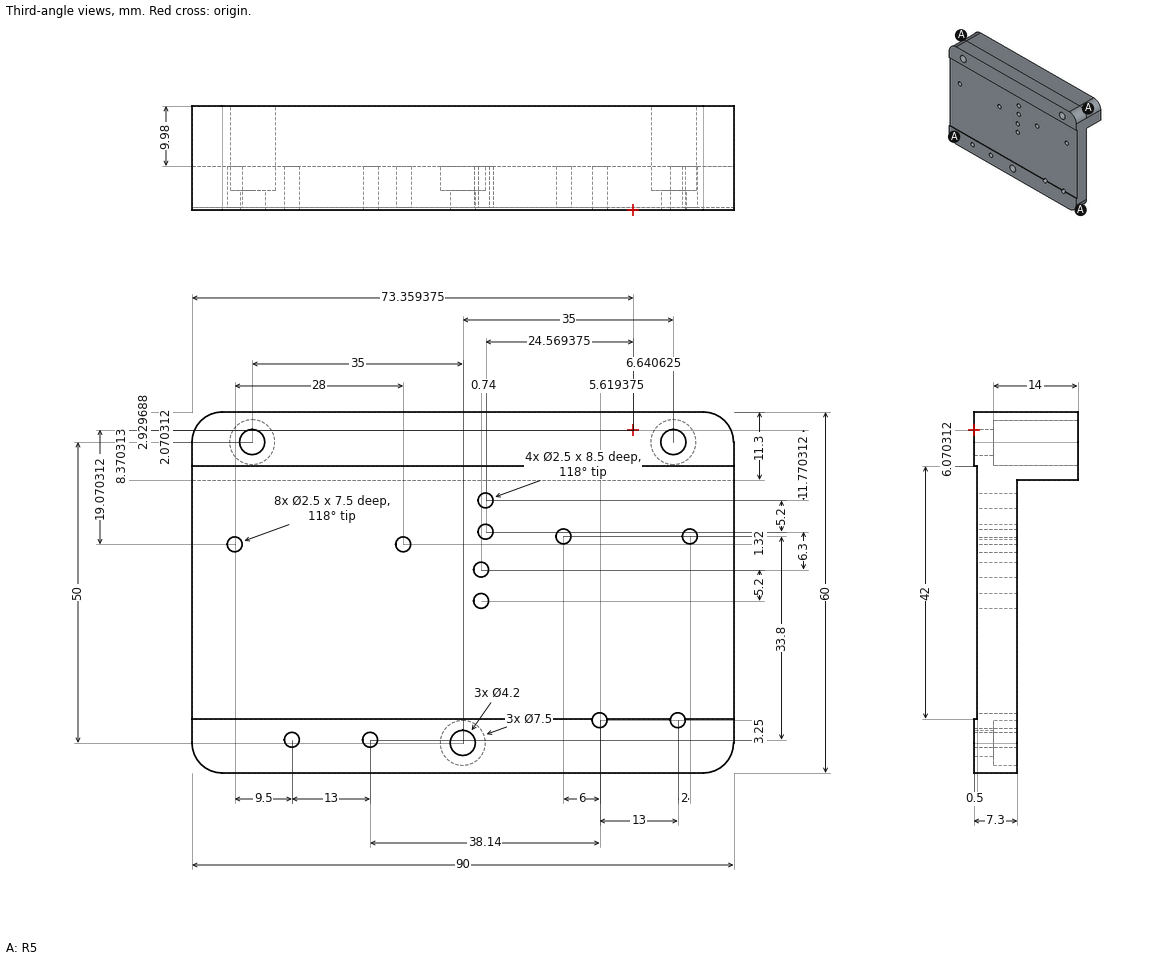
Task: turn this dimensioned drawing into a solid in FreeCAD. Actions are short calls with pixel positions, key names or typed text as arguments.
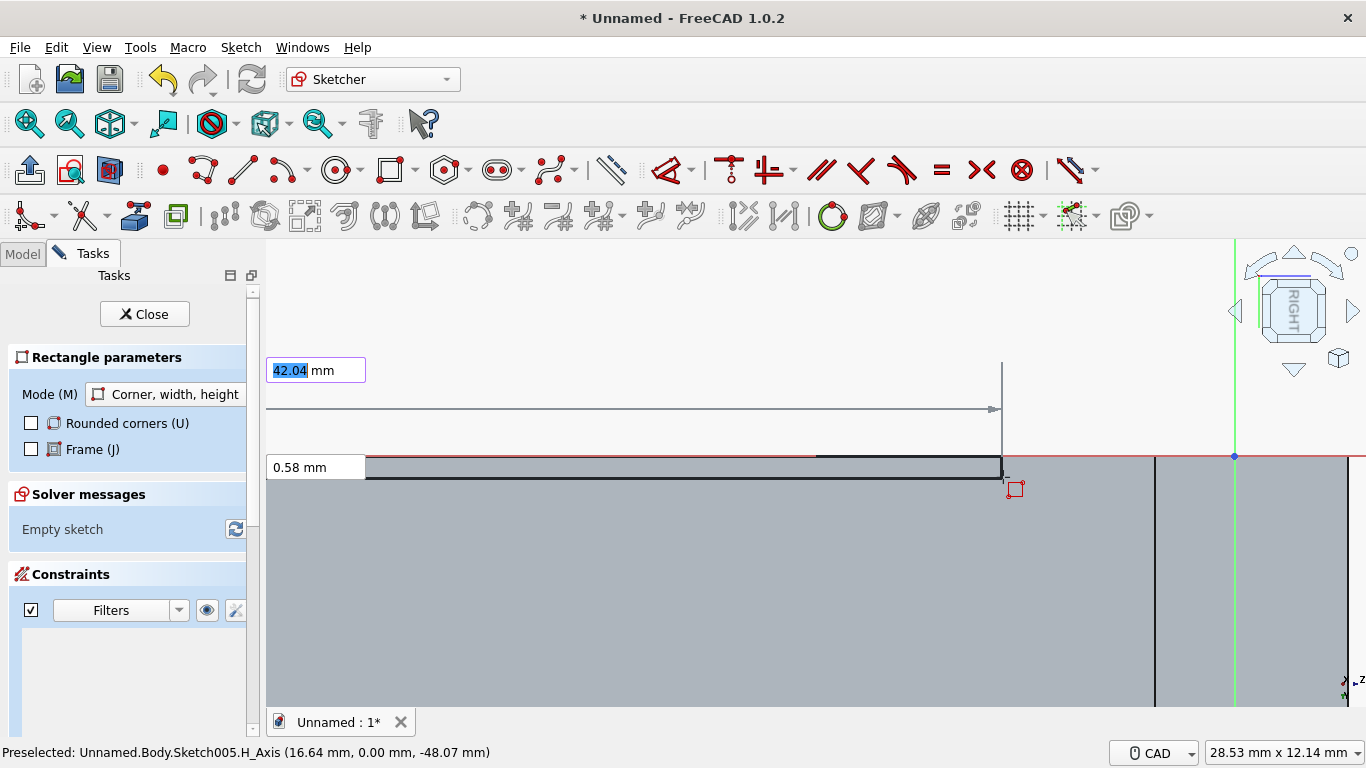
click(1001, 476)
key(Escape)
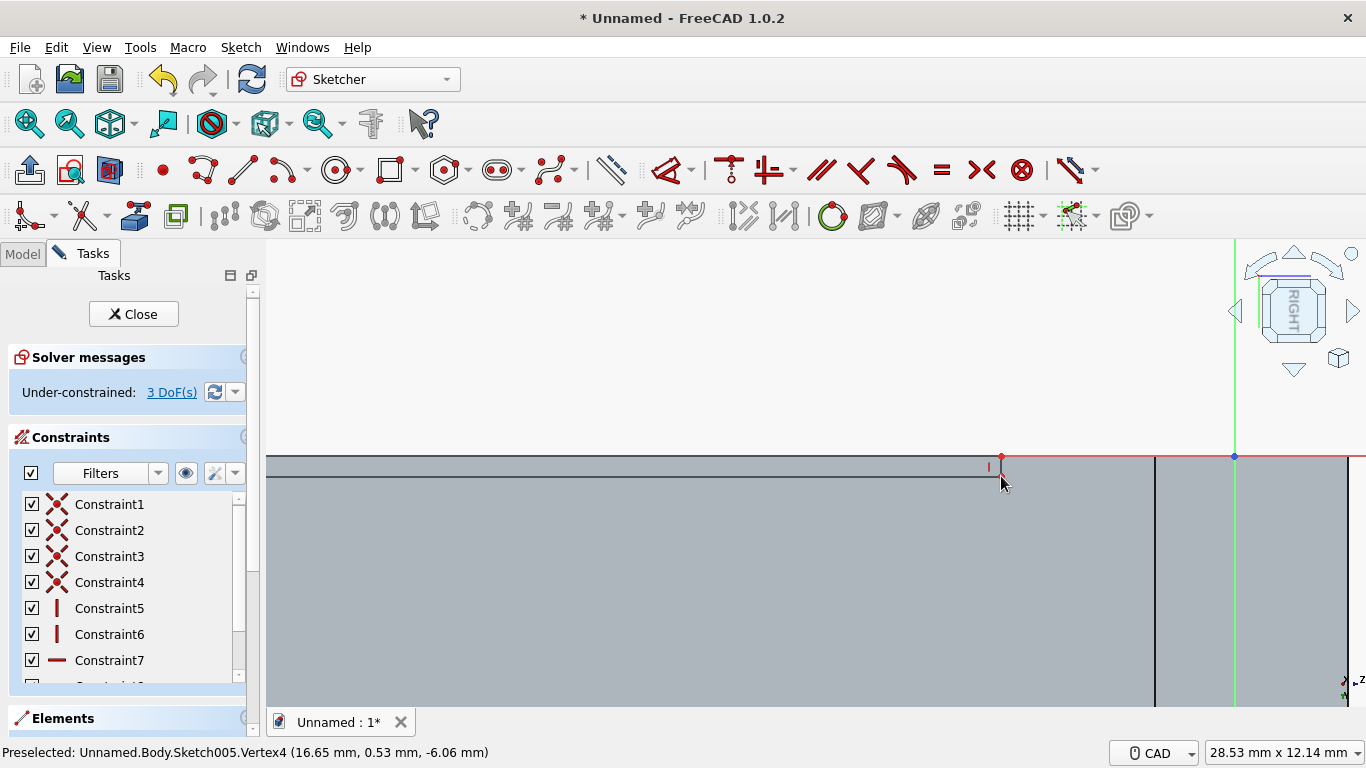
click(666, 170)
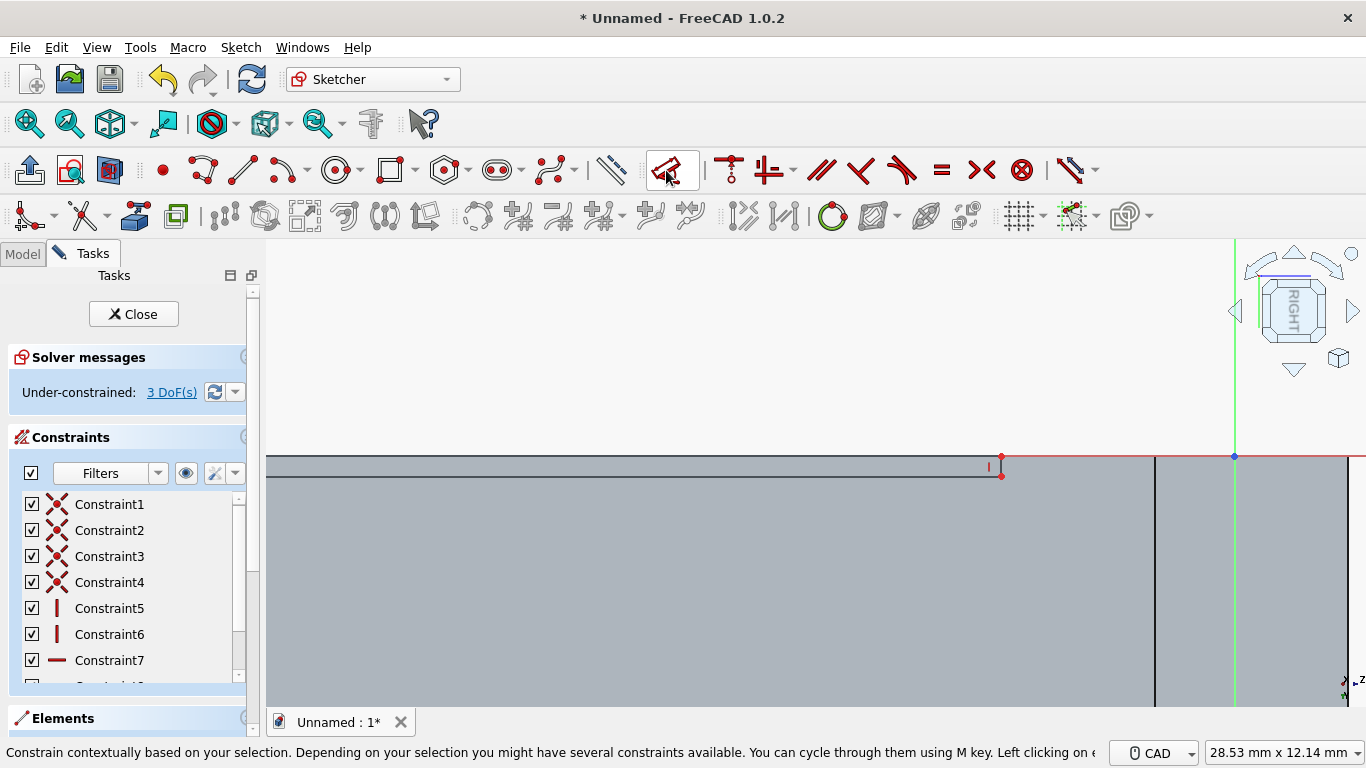
click(515, 477)
click(648, 511)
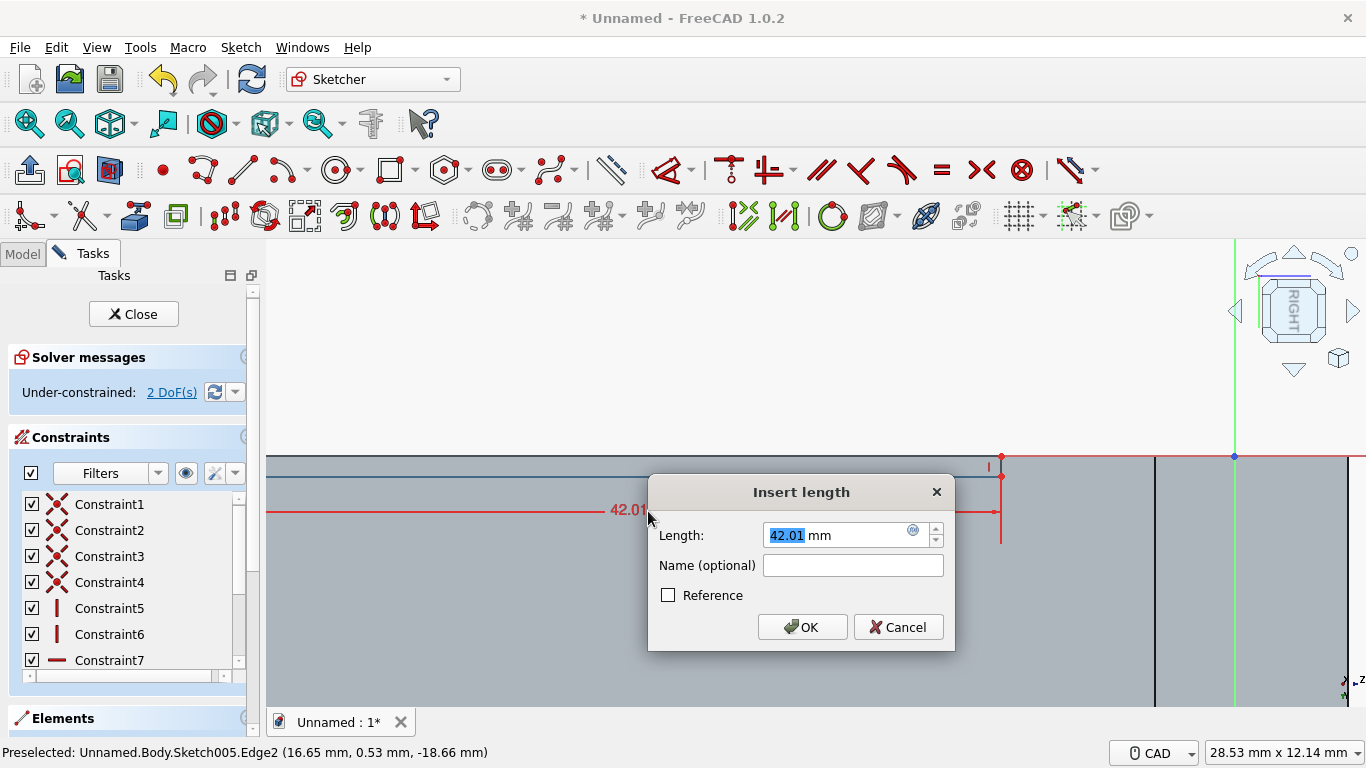
text(42)
key(Return)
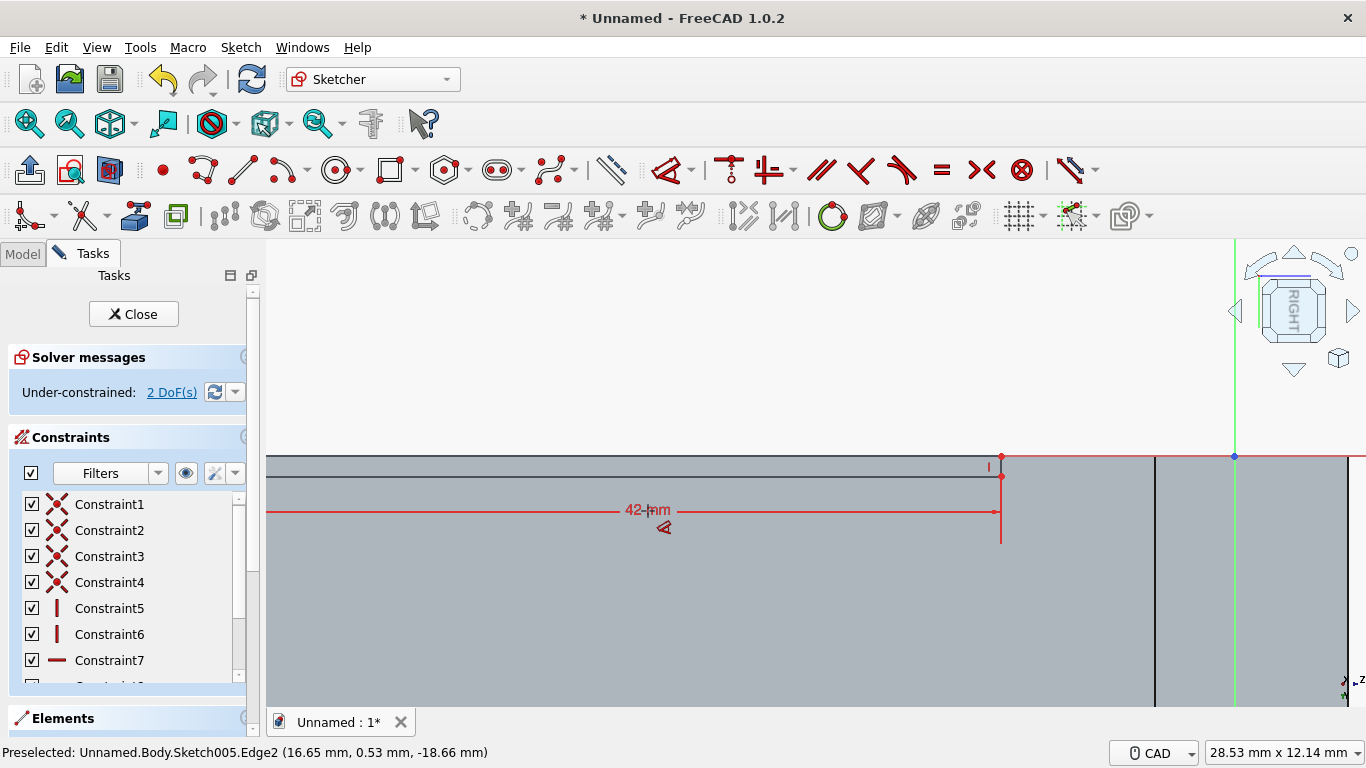
scroll(1003, 477, down, 5)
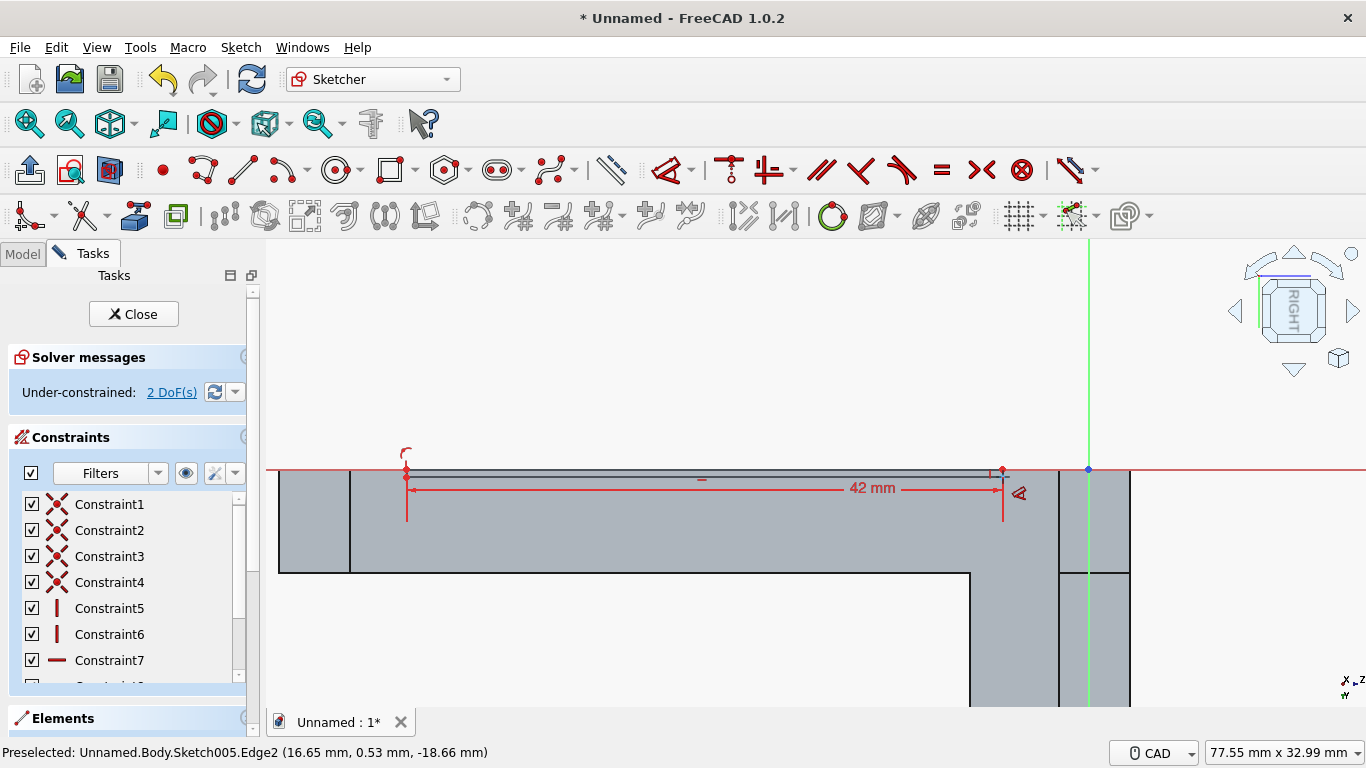
scroll(407, 474, up, 9)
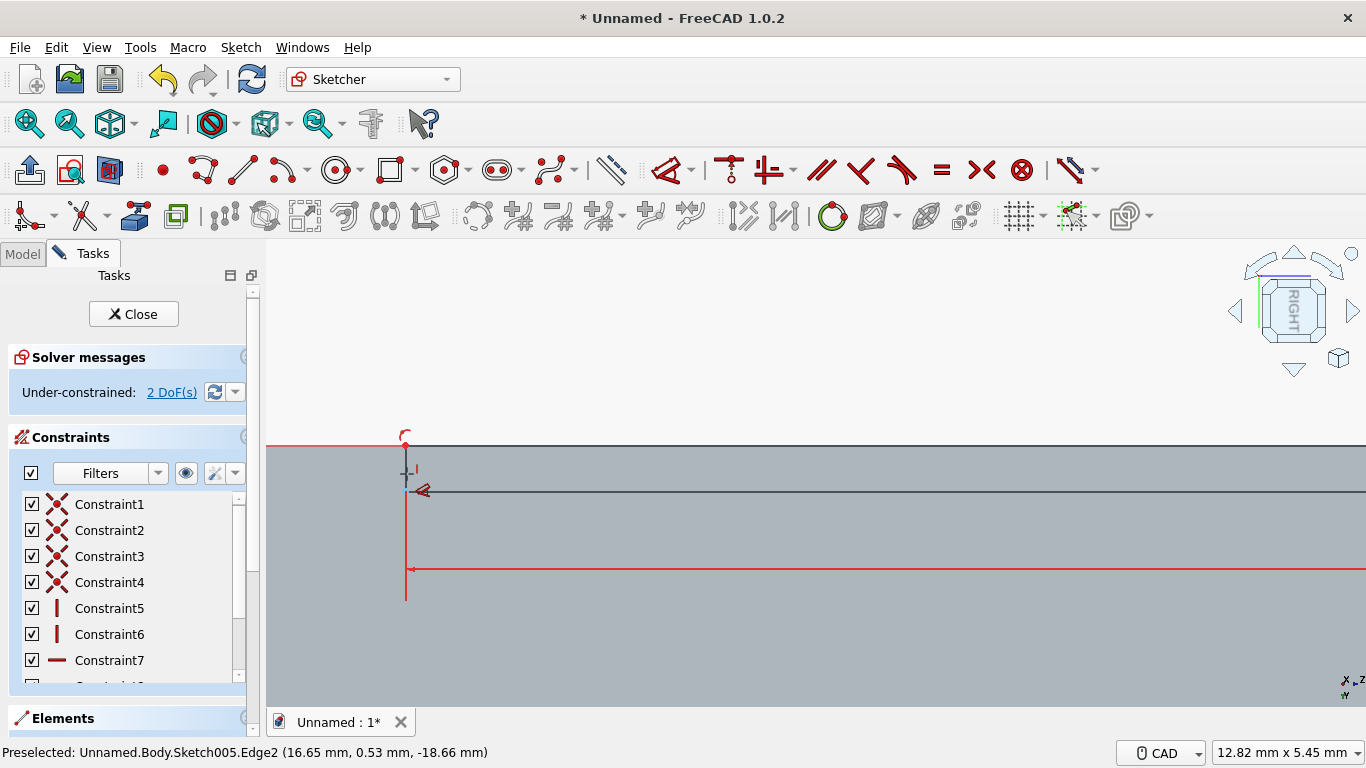
click(406, 469)
click(372, 469)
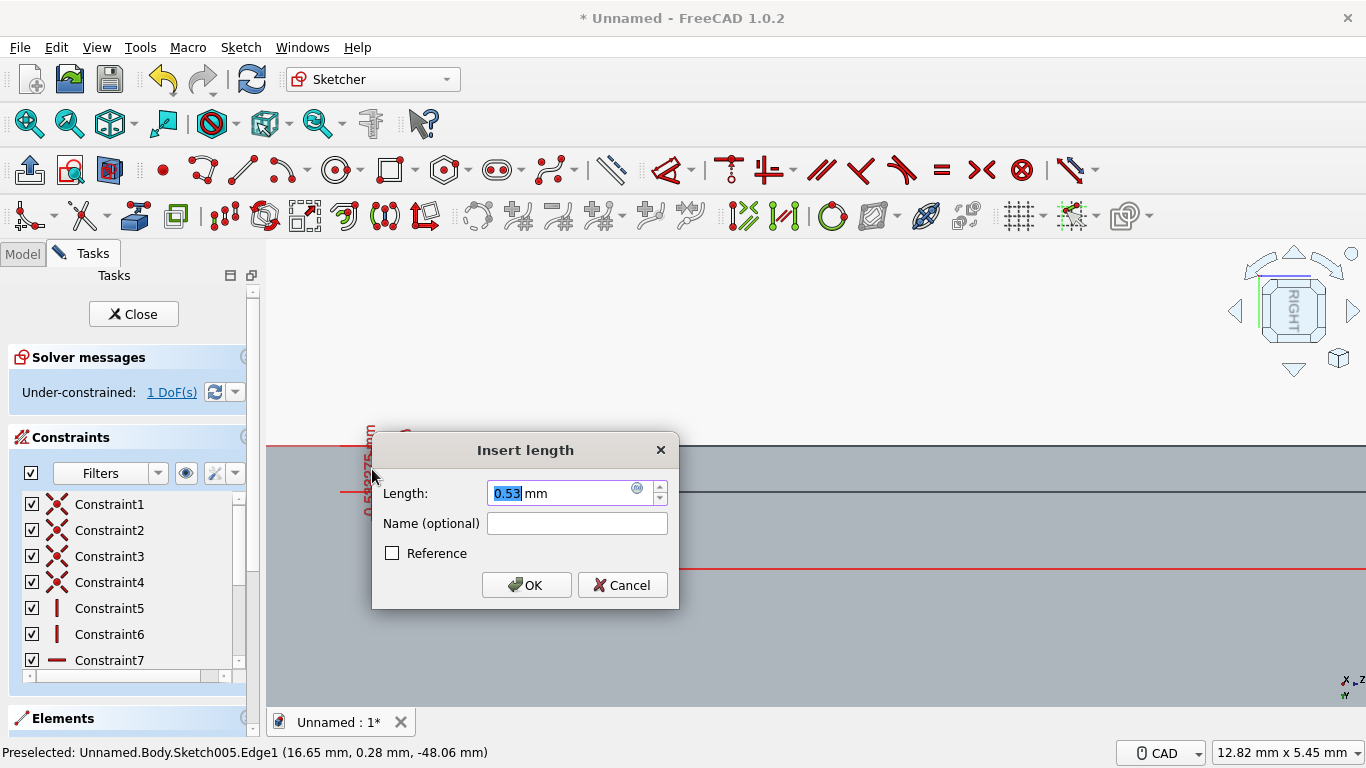
text(0.5)
key(Return)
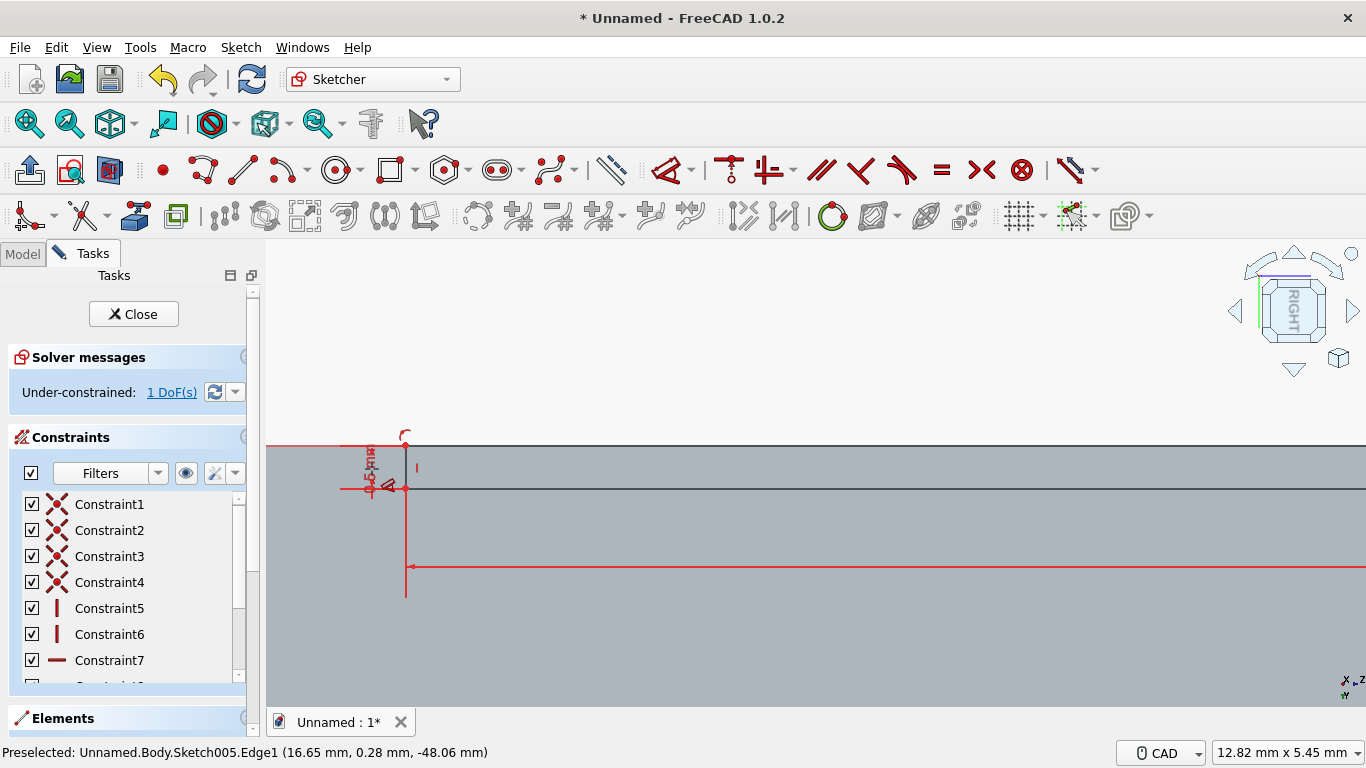
scroll(407, 474, down, 9)